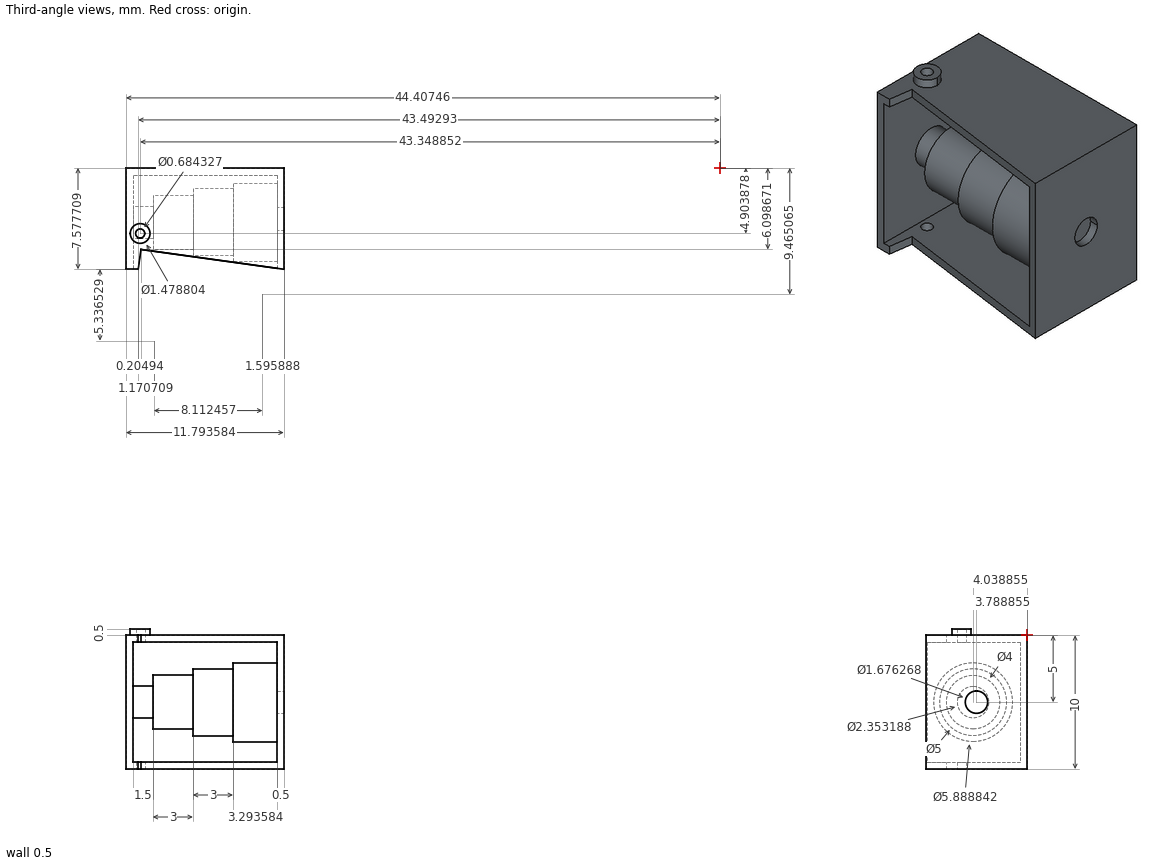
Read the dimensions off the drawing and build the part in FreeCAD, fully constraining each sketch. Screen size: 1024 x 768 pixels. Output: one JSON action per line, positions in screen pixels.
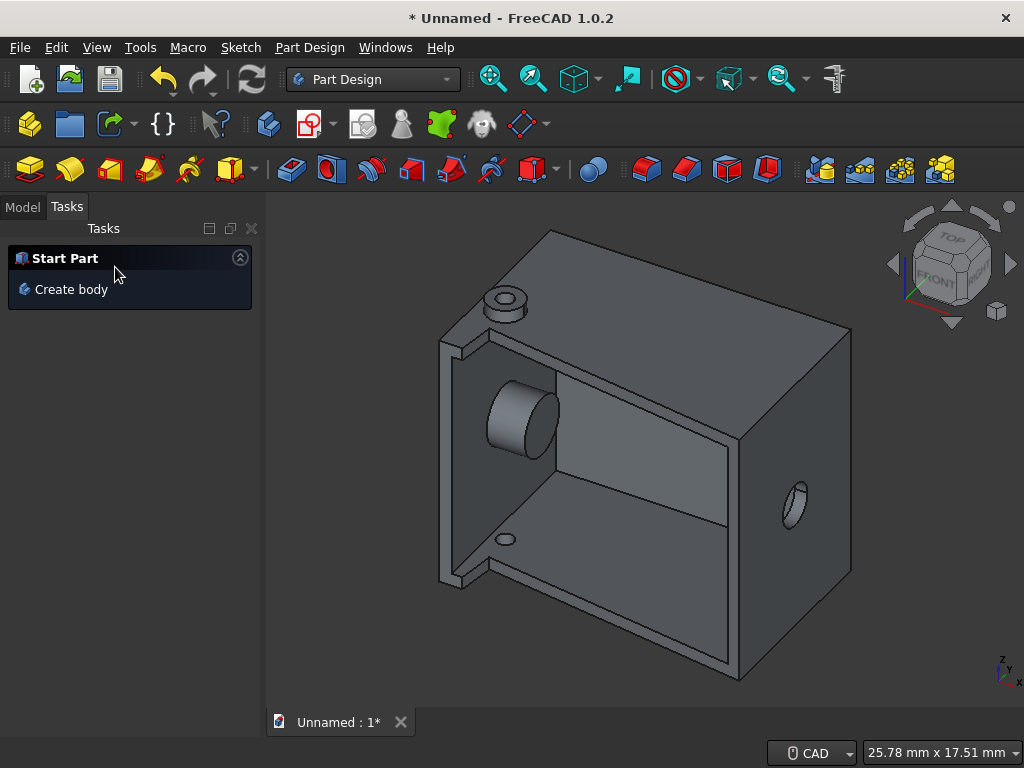
{"action": "left_click", "coordinate": [542, 425]}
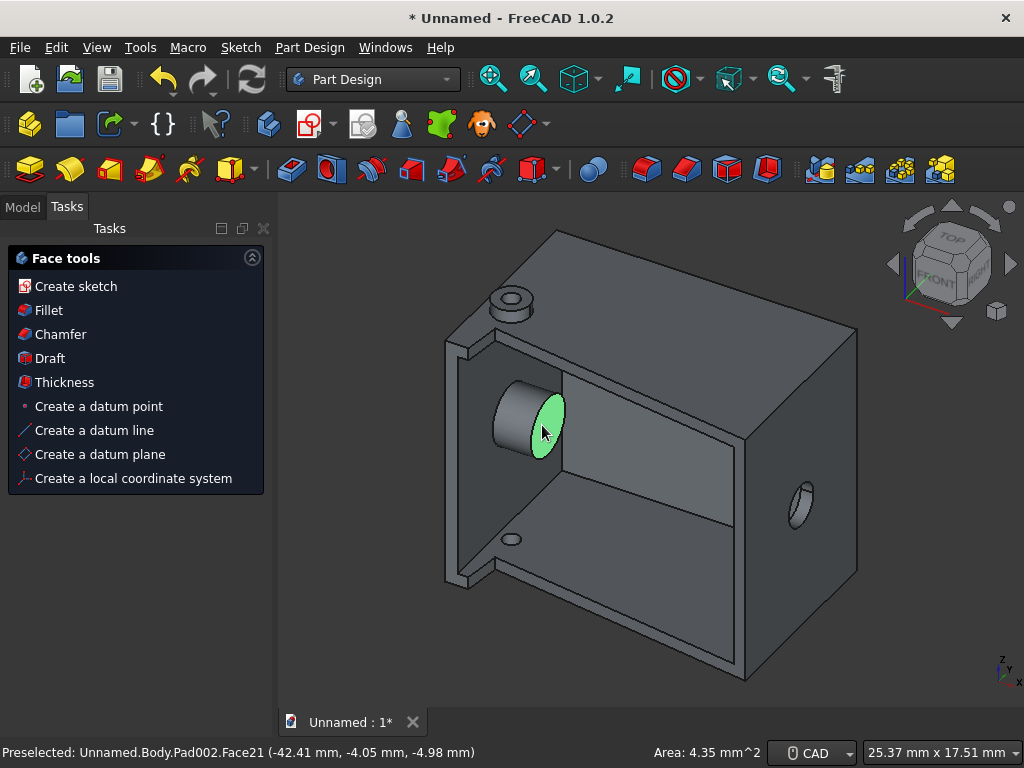
{"action": "left_click", "coordinate": [310, 124]}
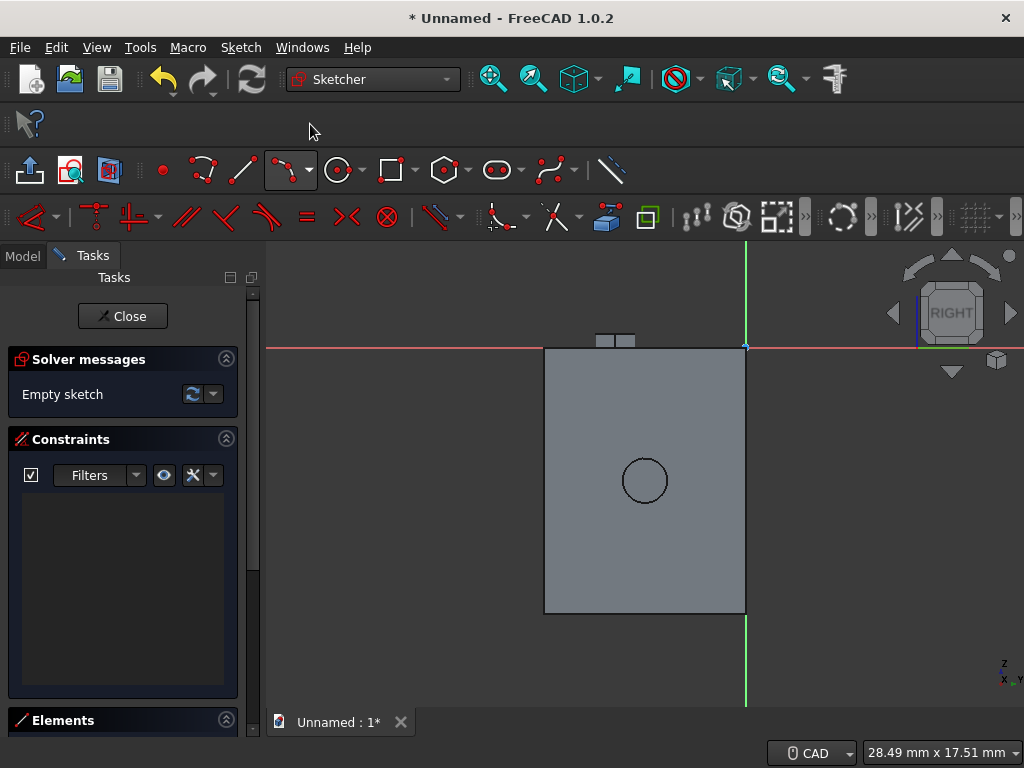
{"action": "left_click", "coordinate": [110, 170]}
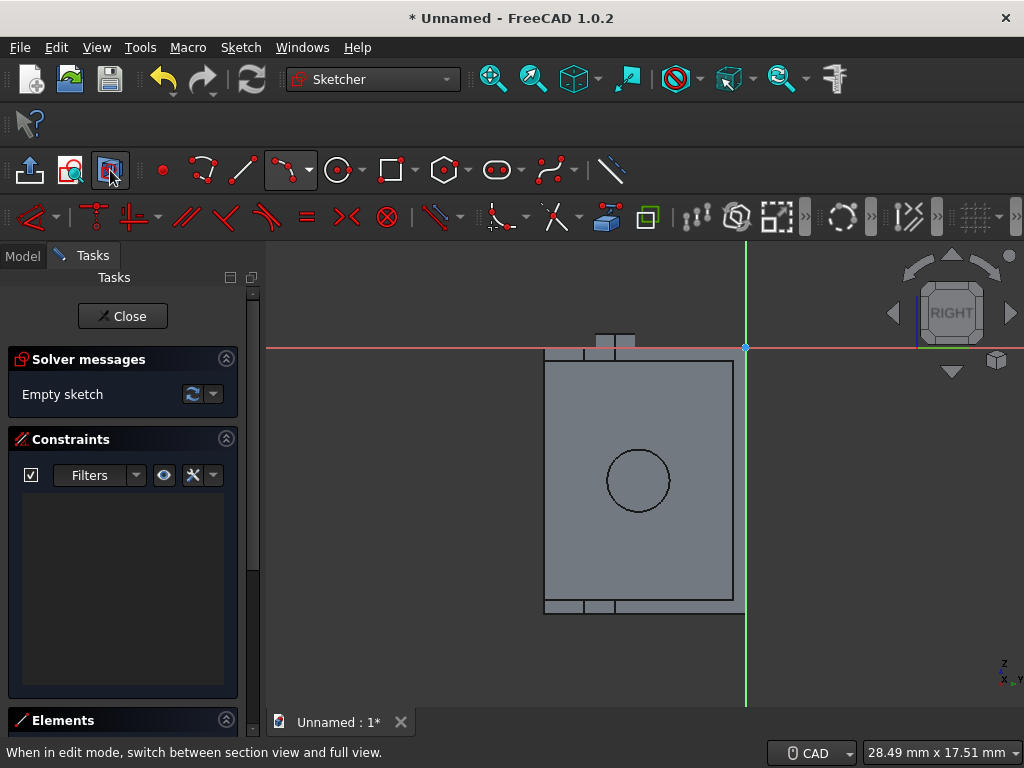
{"action": "scroll", "coordinate": [846, 373], "scroll_direction": "up", "scroll_amount": 2}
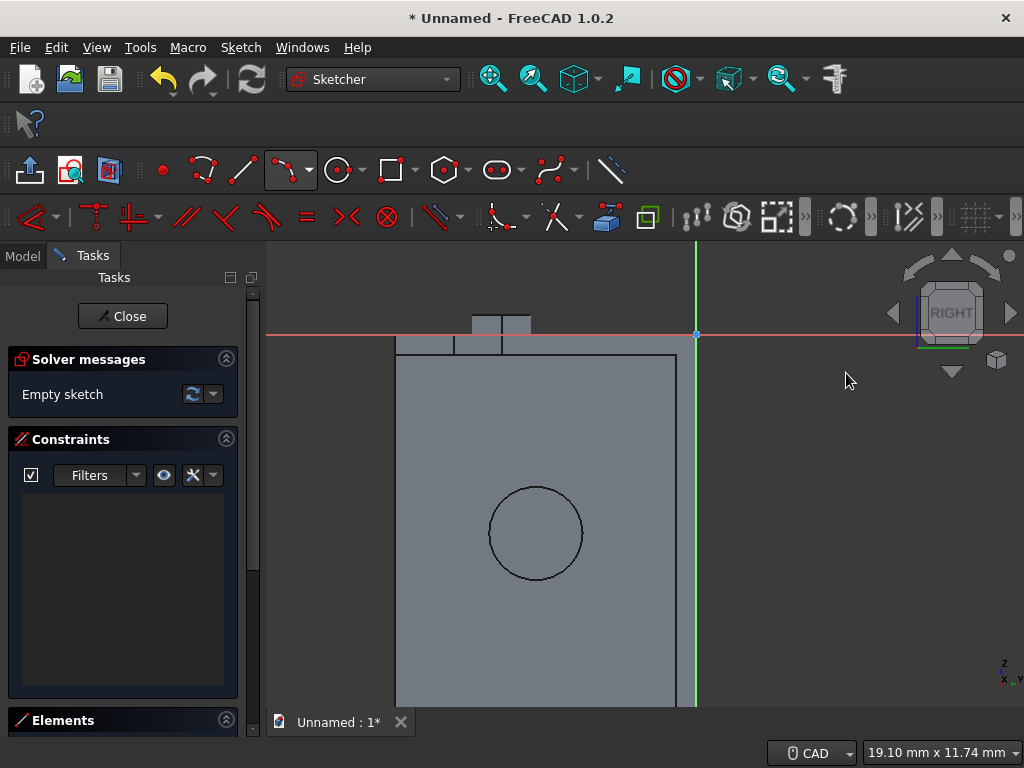
{"action": "left_click", "coordinate": [338, 170]}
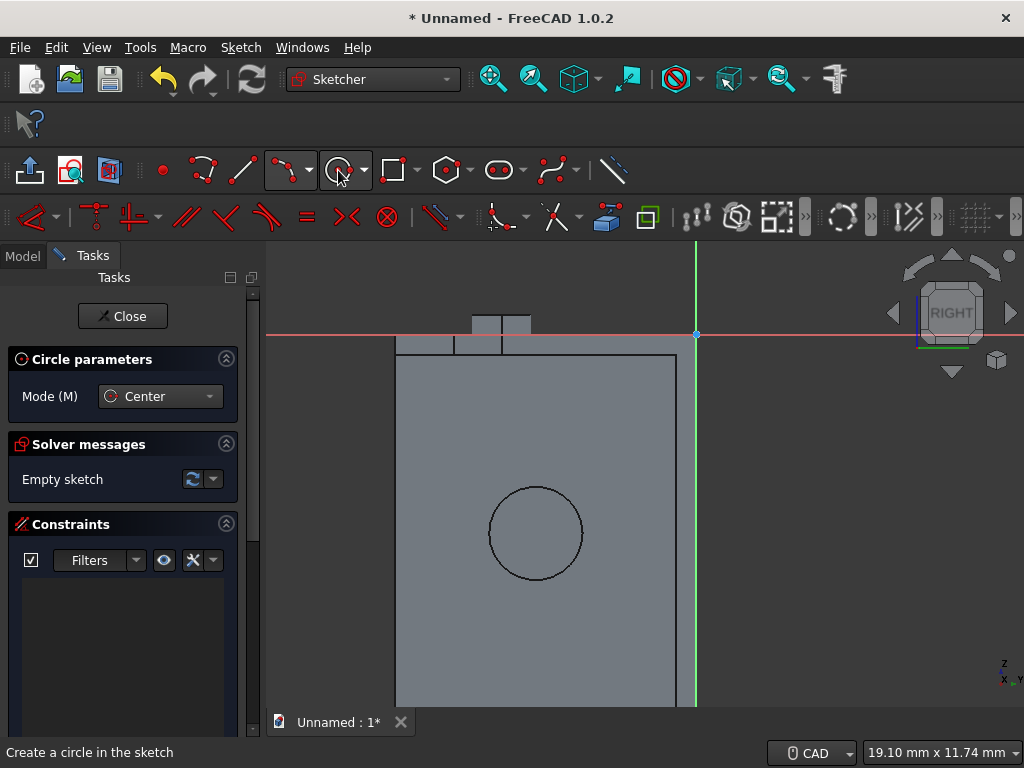
{"action": "left_click", "coordinate": [536, 533]}
{"action": "left_click", "coordinate": [592, 477]}
{"action": "key", "text": "Escape"}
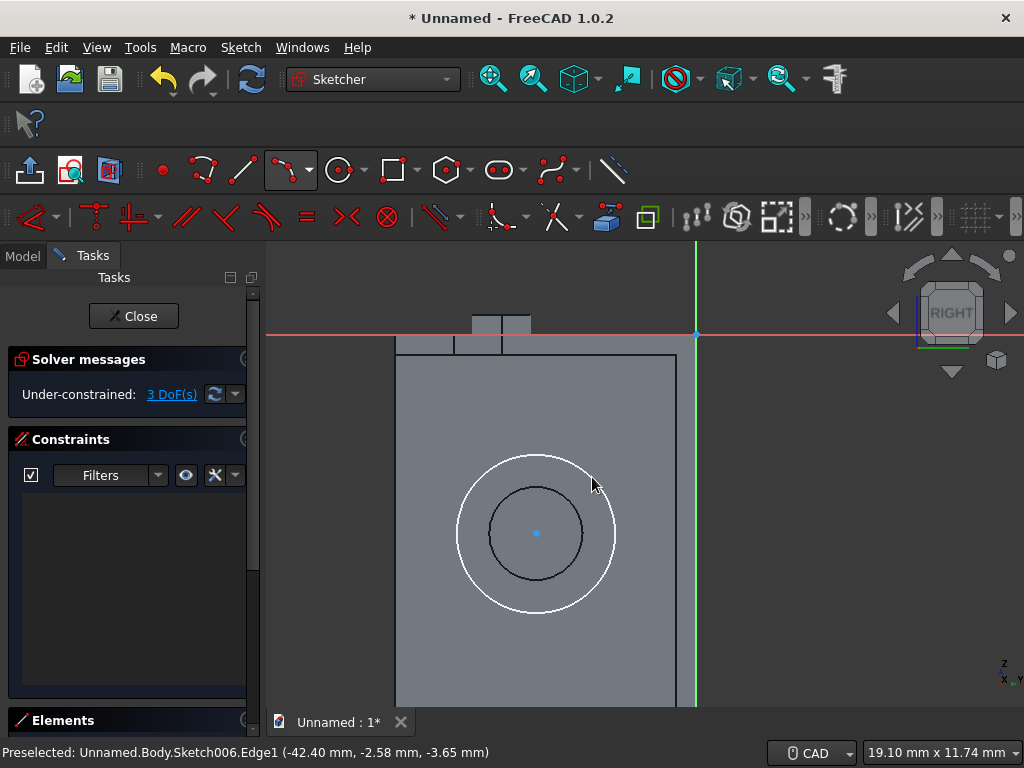
{"action": "left_click", "coordinate": [32, 218]}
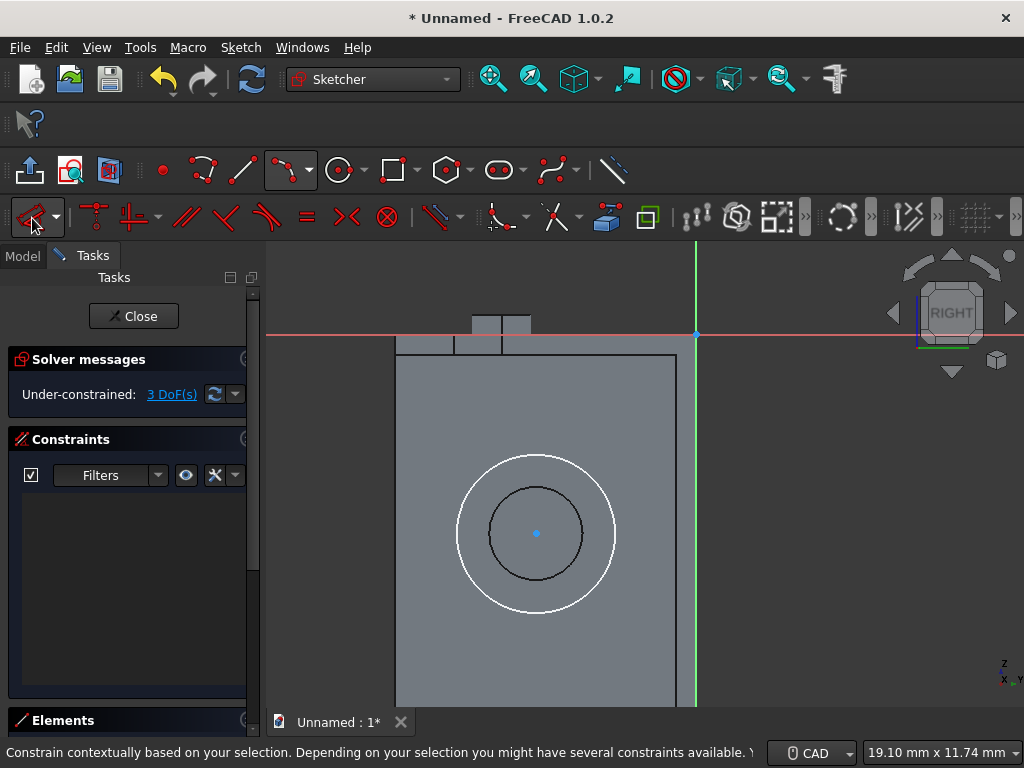
{"action": "left_click", "coordinate": [592, 478]}
{"action": "left_click", "coordinate": [615, 455]}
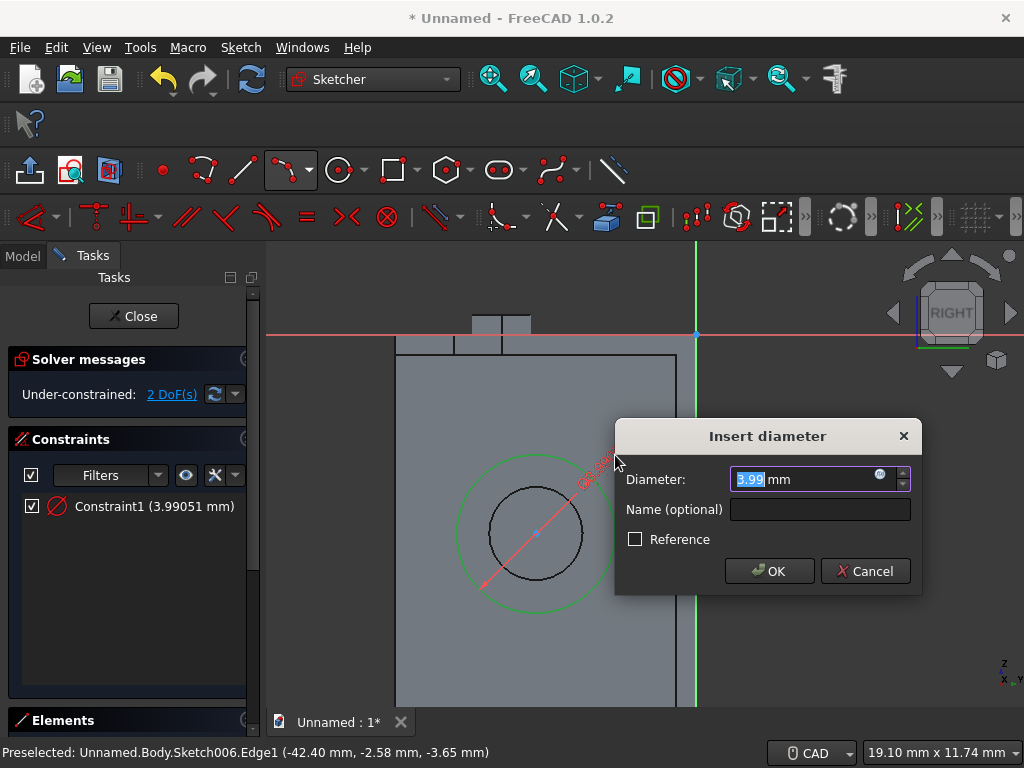
{"action": "type", "text": "4"}
{"action": "key", "text": "Return"}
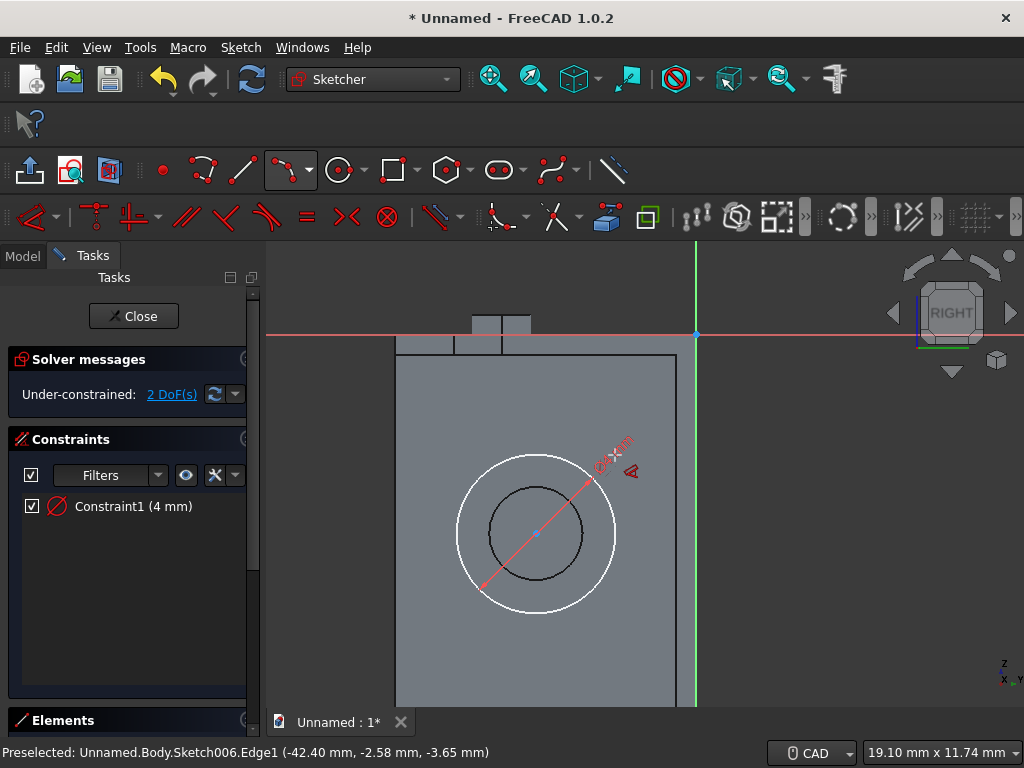
{"action": "left_click", "coordinate": [536, 534]}
{"action": "left_click", "coordinate": [730, 434]}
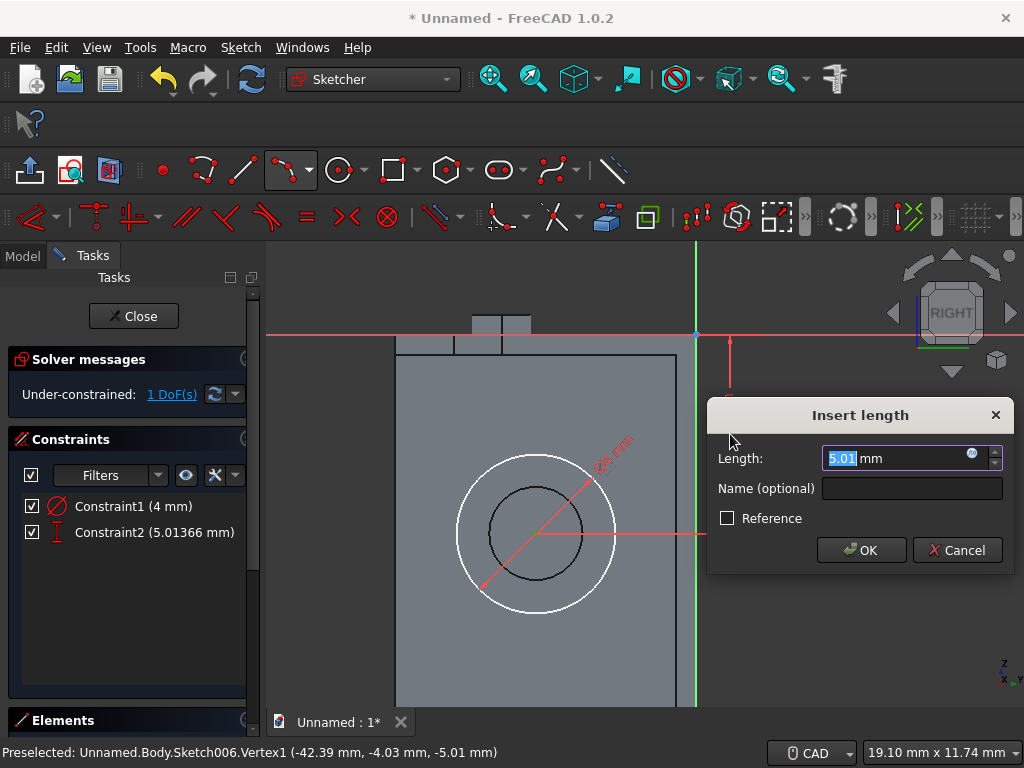
{"action": "type", "text": "5"}
{"action": "key", "text": "Return"}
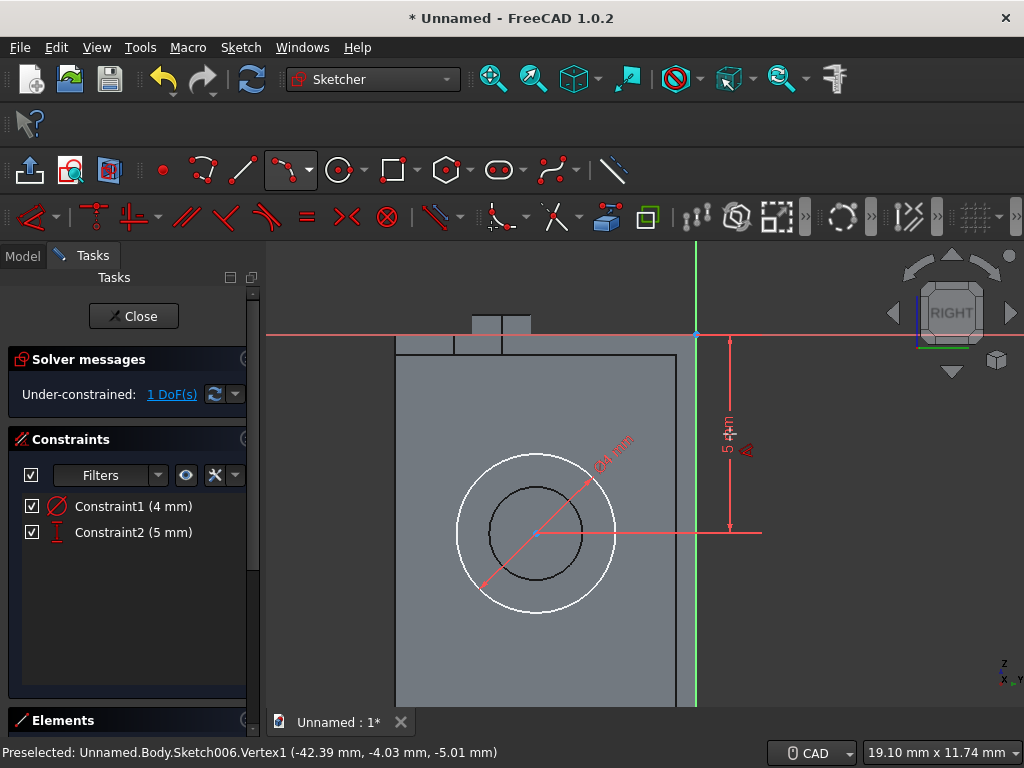
{"action": "left_click", "coordinate": [536, 533]}
{"action": "left_click", "coordinate": [616, 301]}